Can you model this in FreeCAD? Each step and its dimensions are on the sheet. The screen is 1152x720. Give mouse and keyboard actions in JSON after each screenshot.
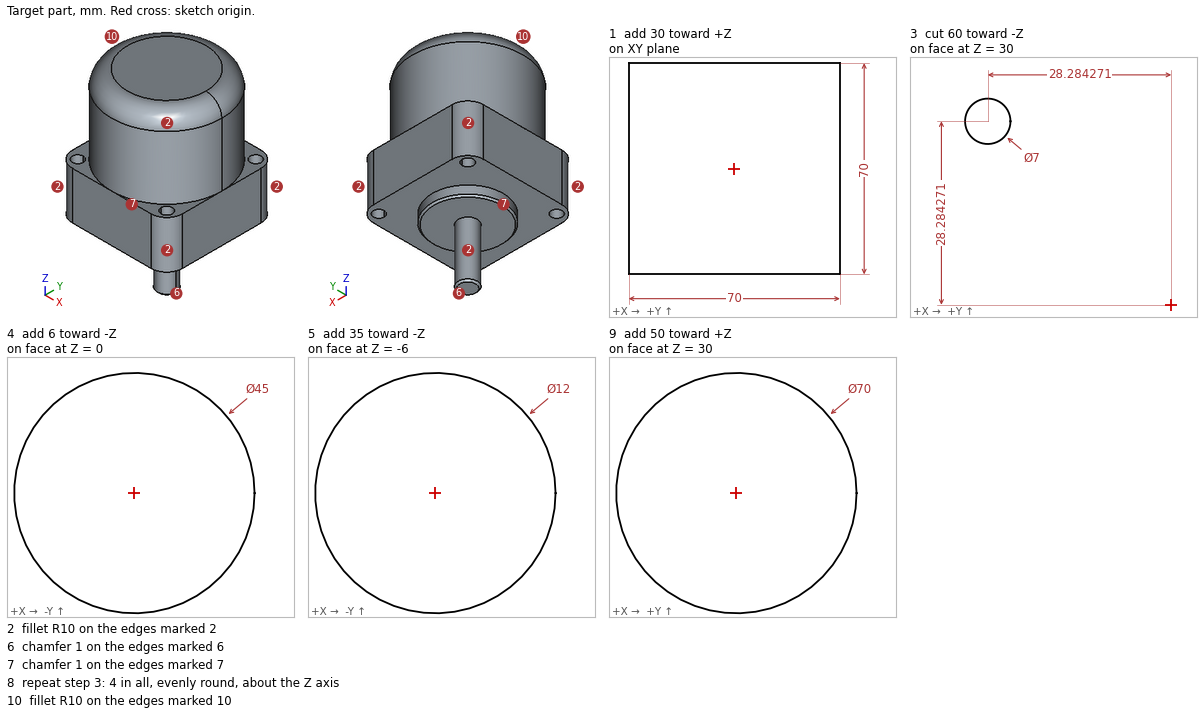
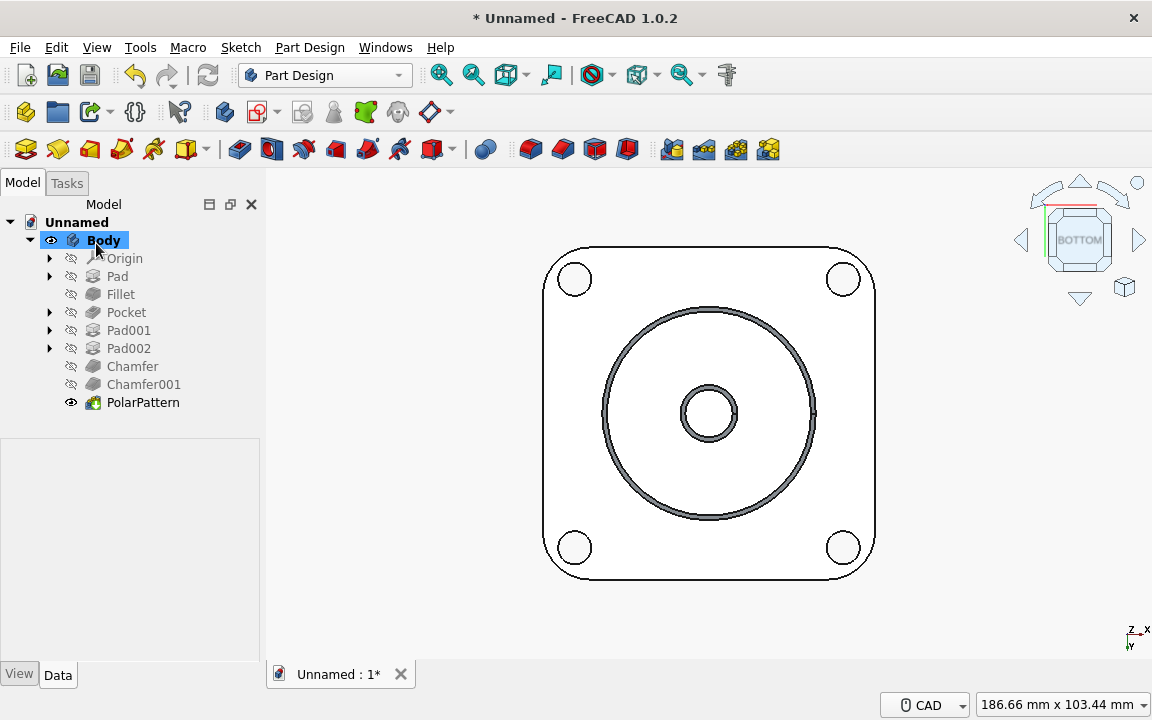
{"action": "key", "text": "0"}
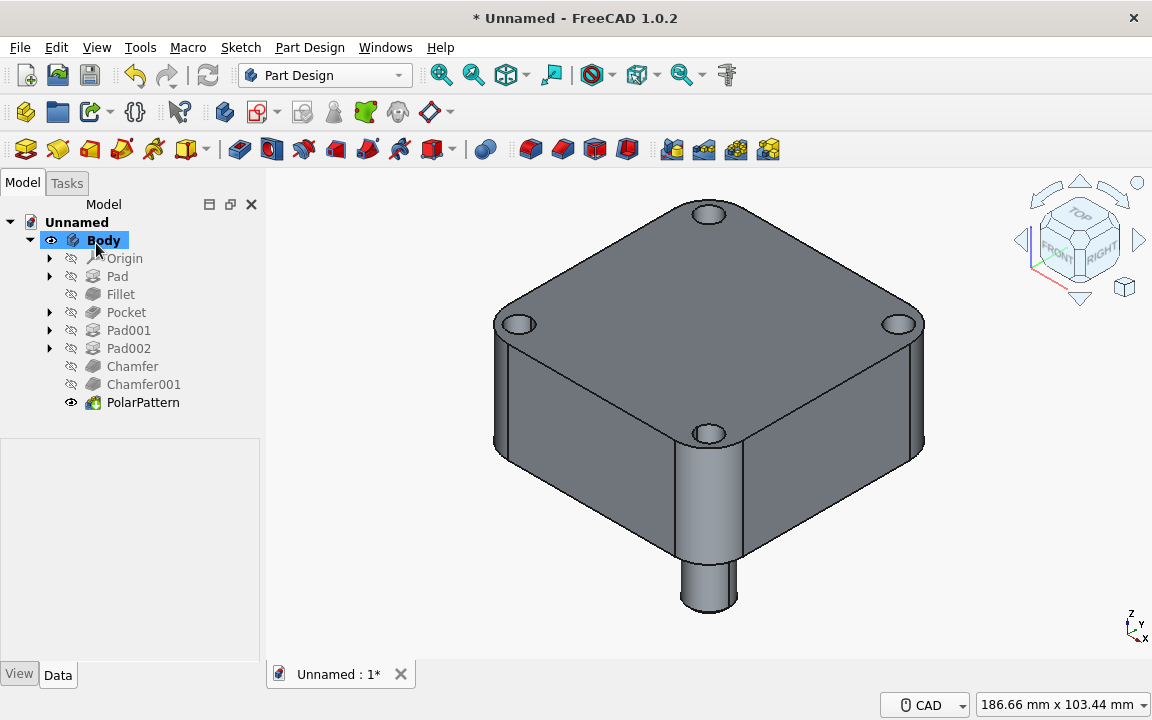
{"action": "left_click", "coordinate": [442, 76]}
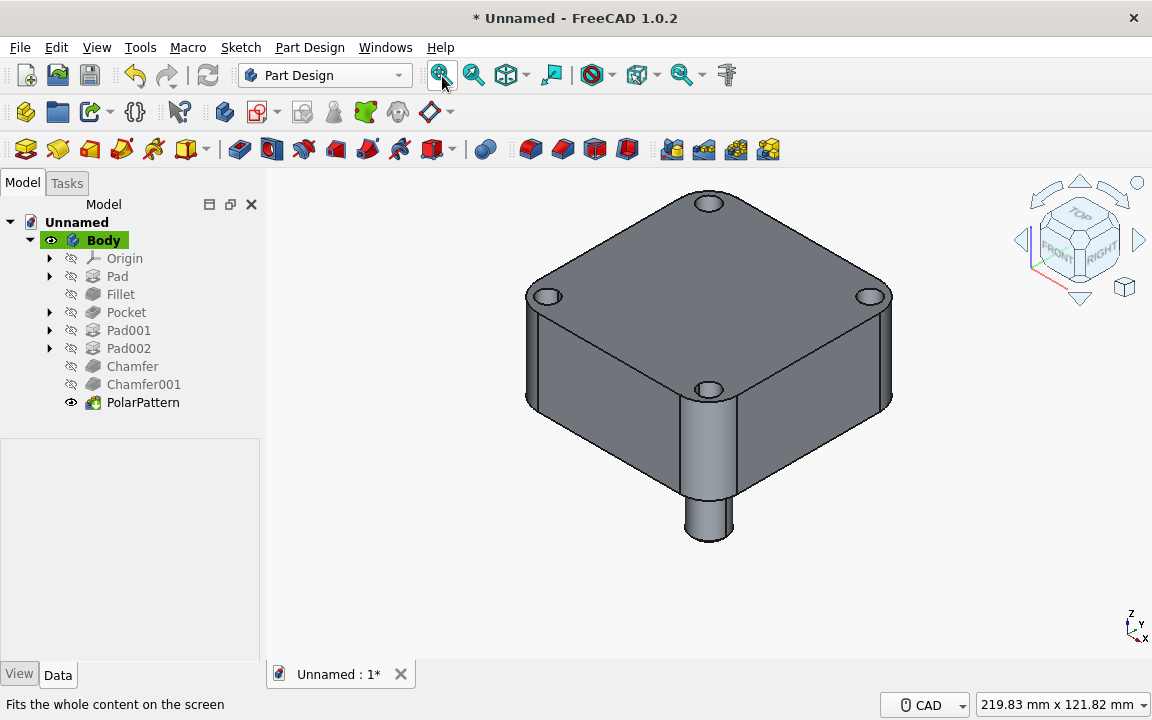
{"action": "left_click", "coordinate": [709, 296]}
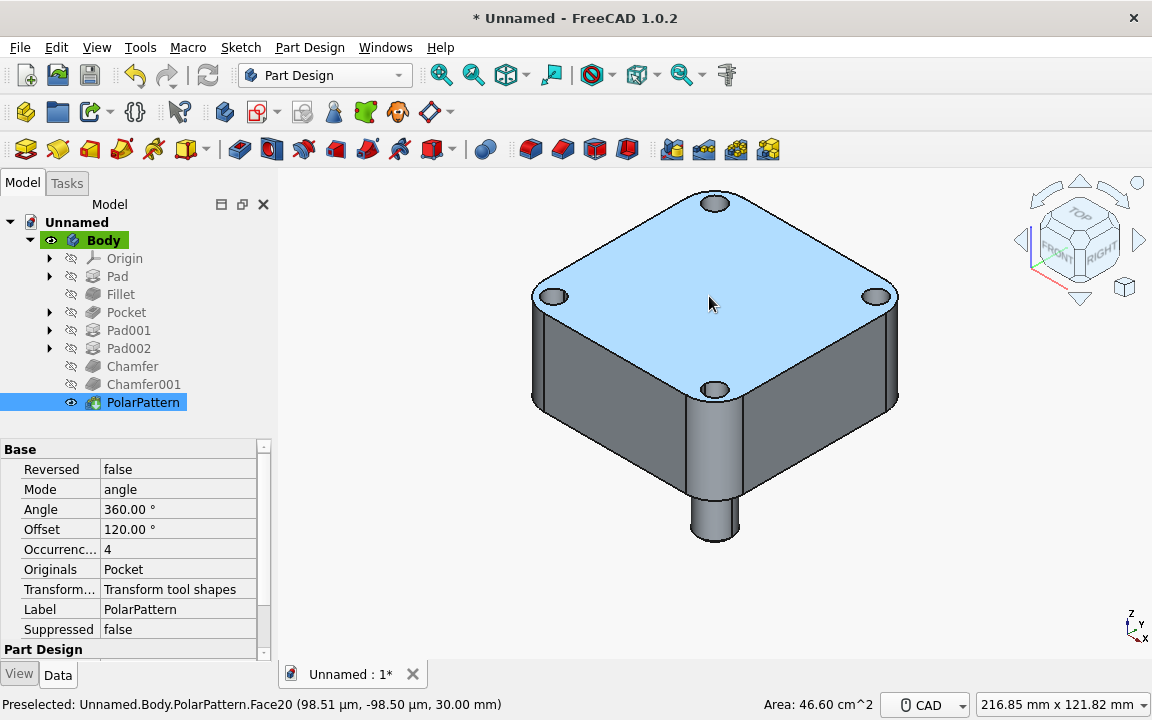
{"action": "left_click", "coordinate": [258, 112]}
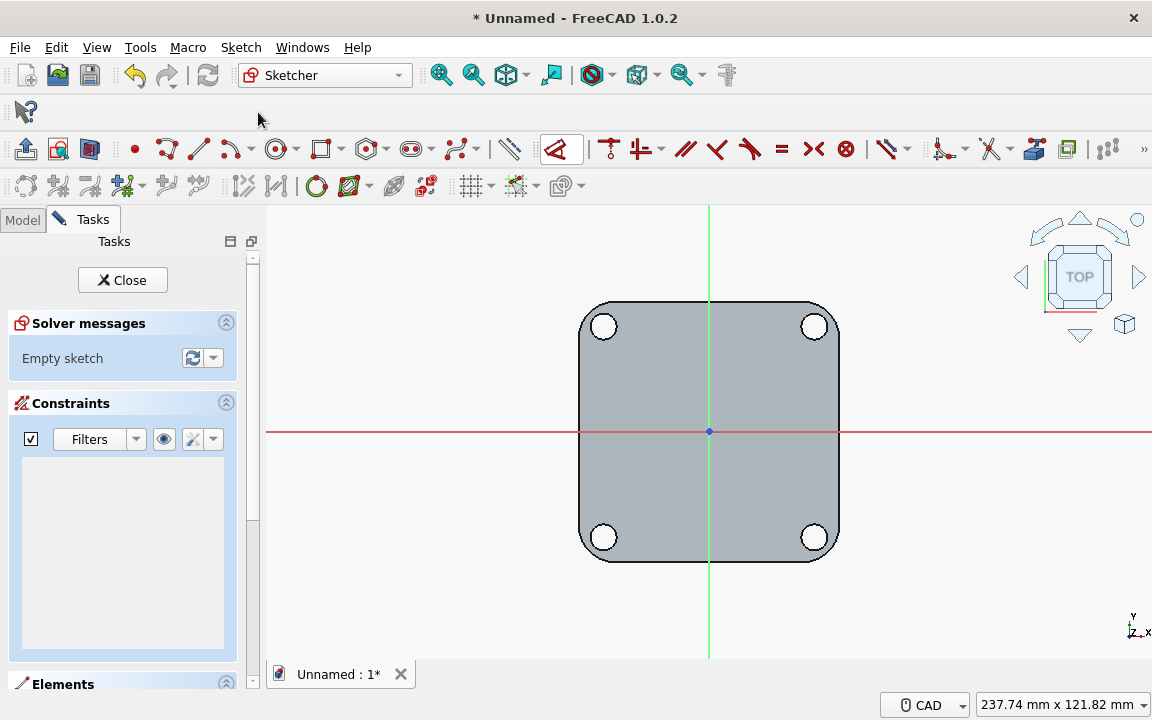
{"action": "key", "text": "g c"}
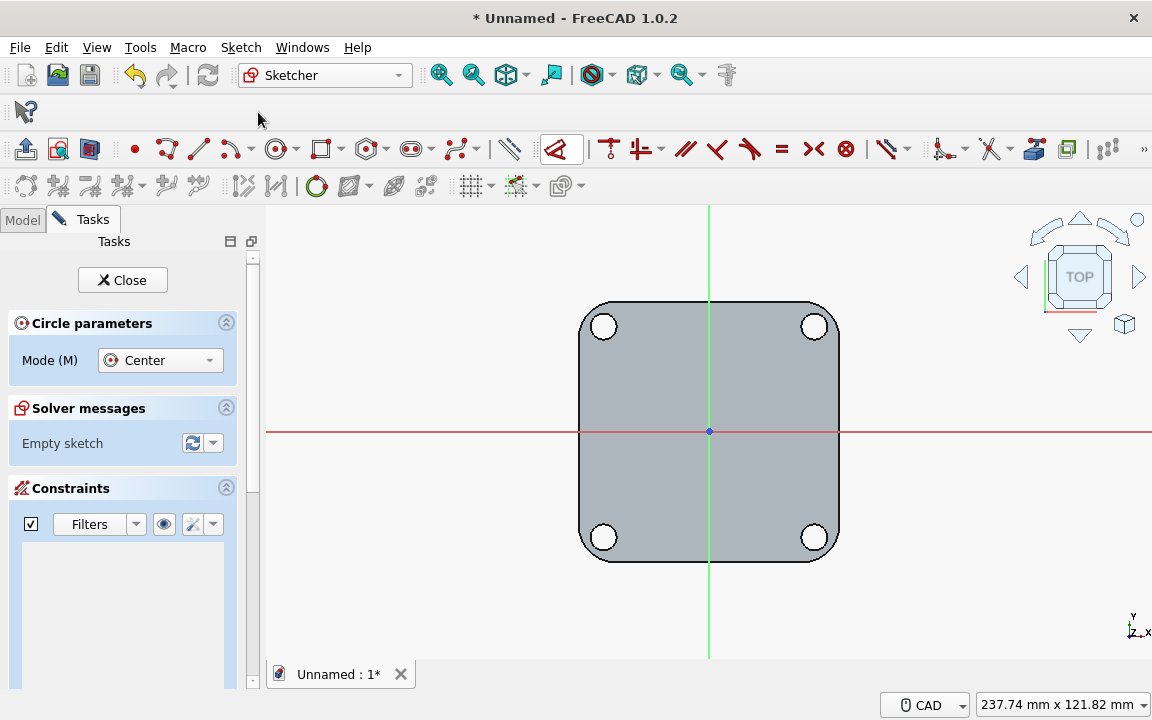
{"action": "left_click", "coordinate": [709, 432]}
{"action": "mouse_move", "coordinate": [801, 340]}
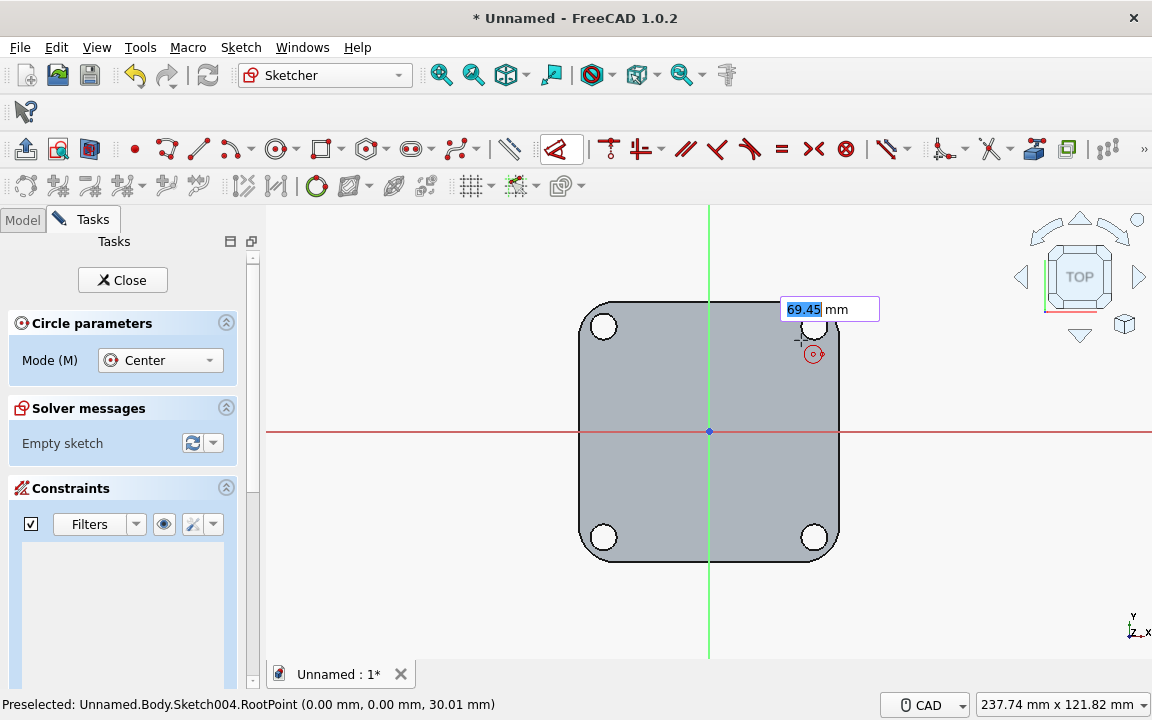
{"action": "type", "text": "70"}
{"action": "key", "text": "Return"}
{"action": "key", "text": "Escape"}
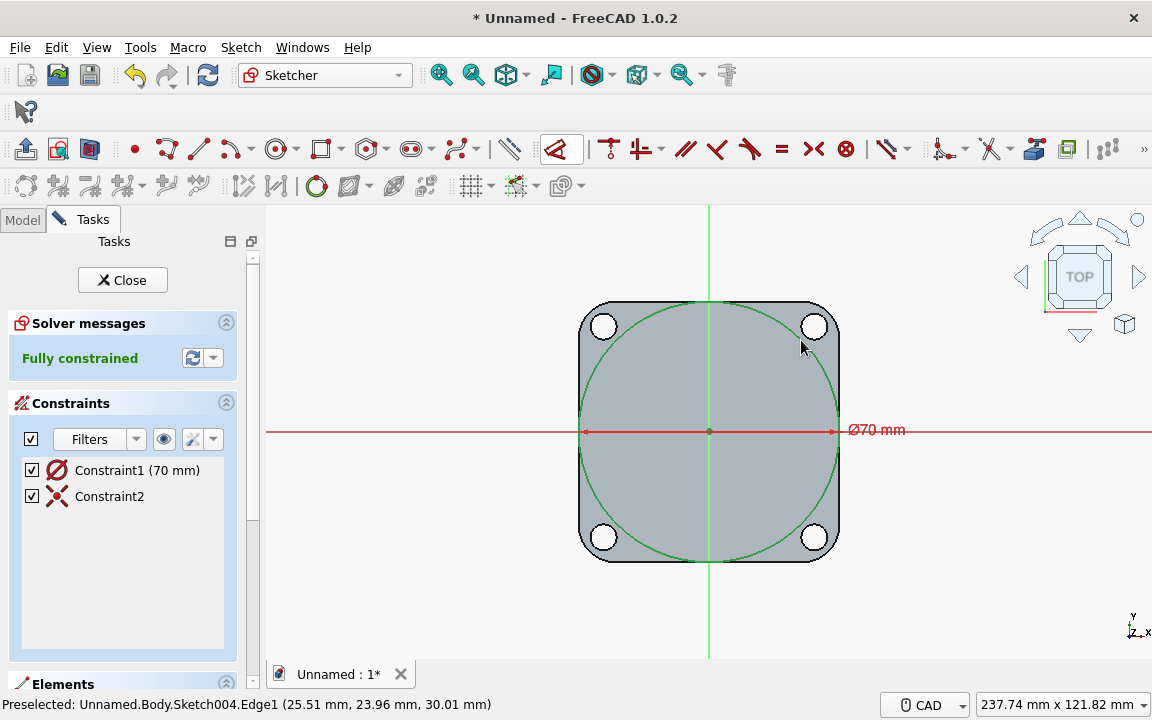
{"action": "left_click", "coordinate": [123, 280]}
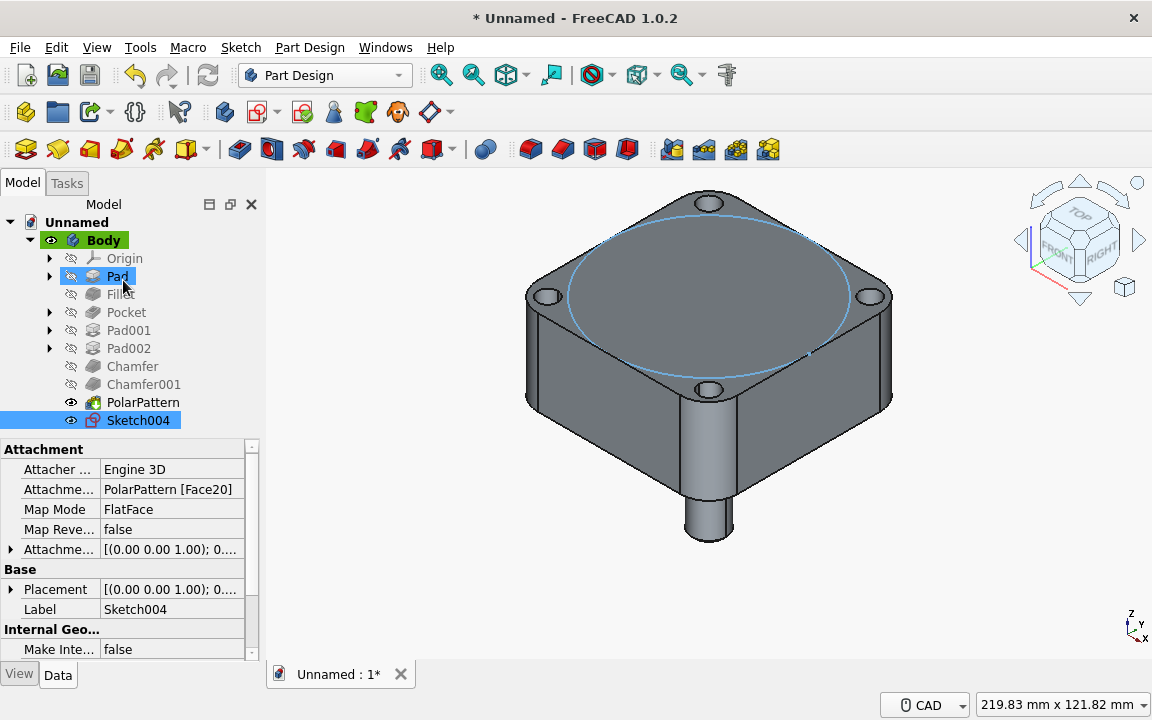
{"action": "left_click", "coordinate": [26, 150]}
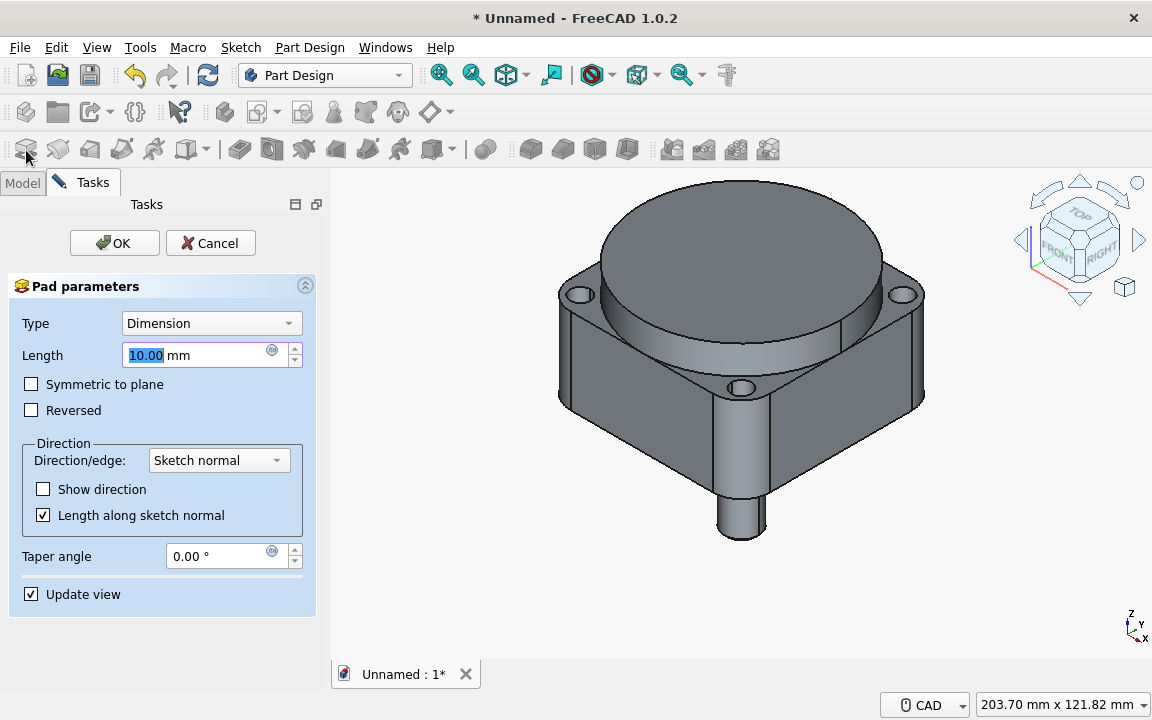
{"action": "type", "text": "50"}
{"action": "key", "text": "Tab"}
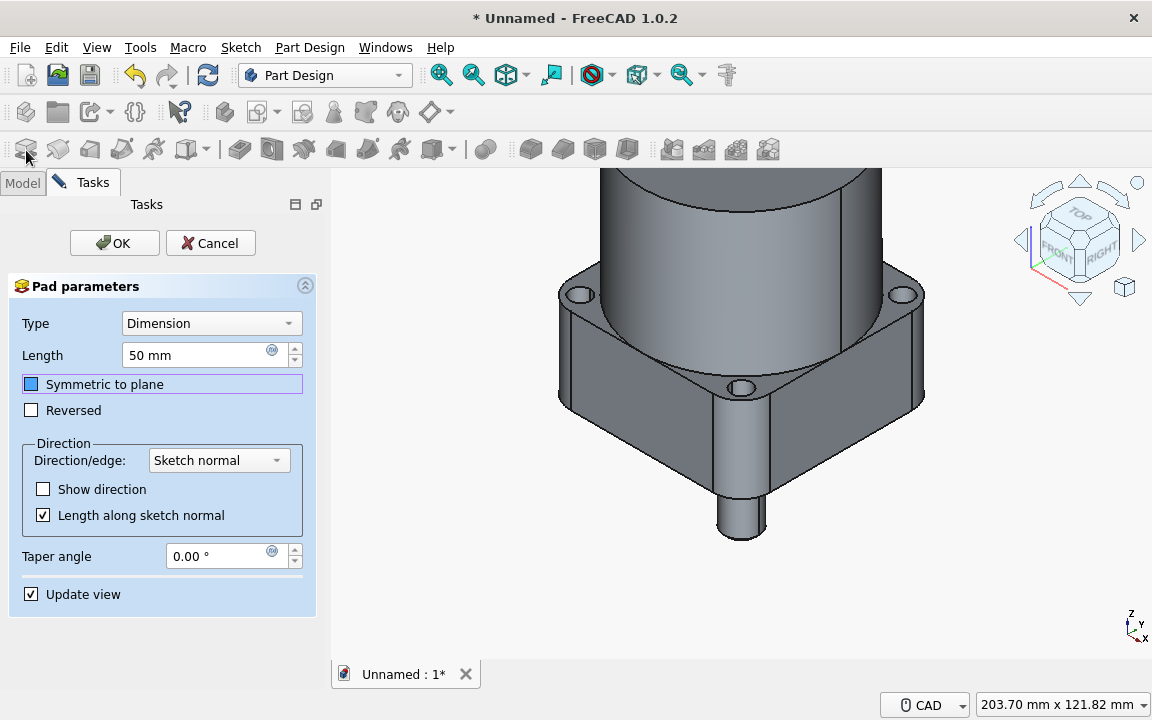
{"action": "left_click", "coordinate": [115, 243]}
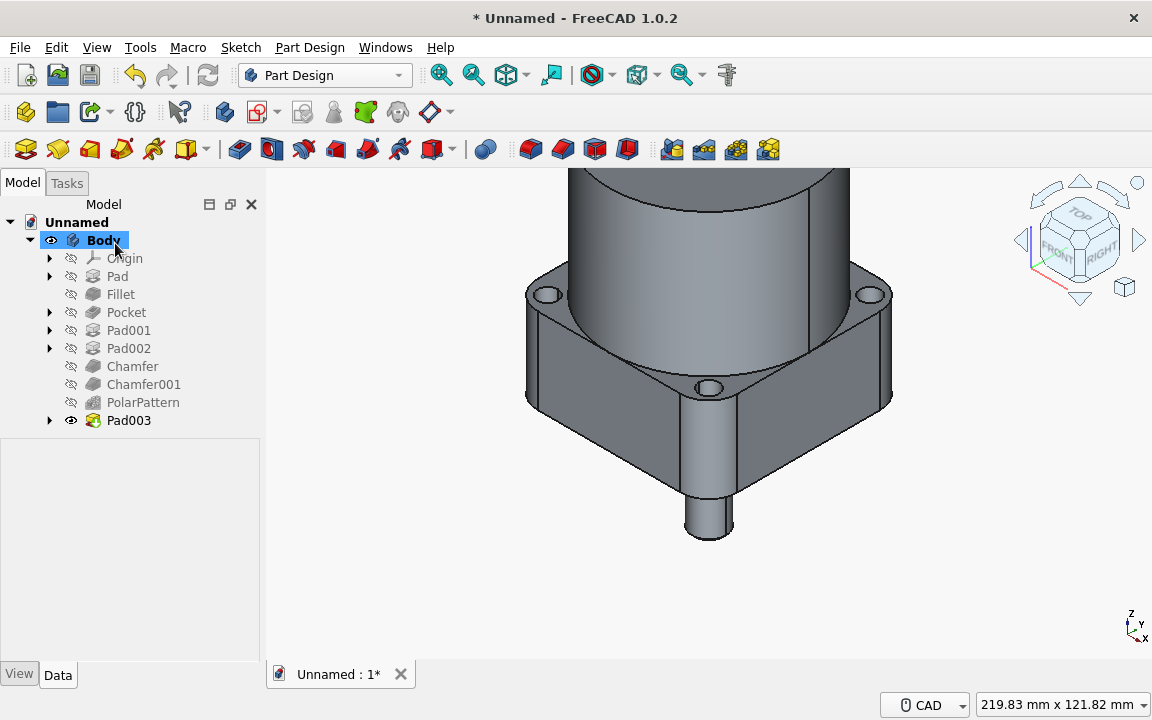
{"action": "key", "text": "v f"}